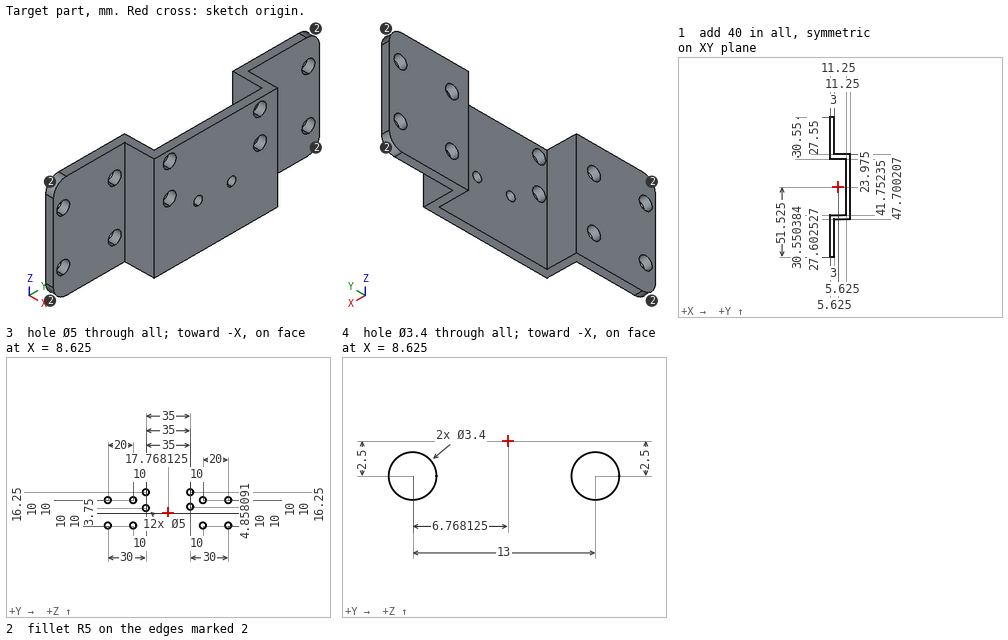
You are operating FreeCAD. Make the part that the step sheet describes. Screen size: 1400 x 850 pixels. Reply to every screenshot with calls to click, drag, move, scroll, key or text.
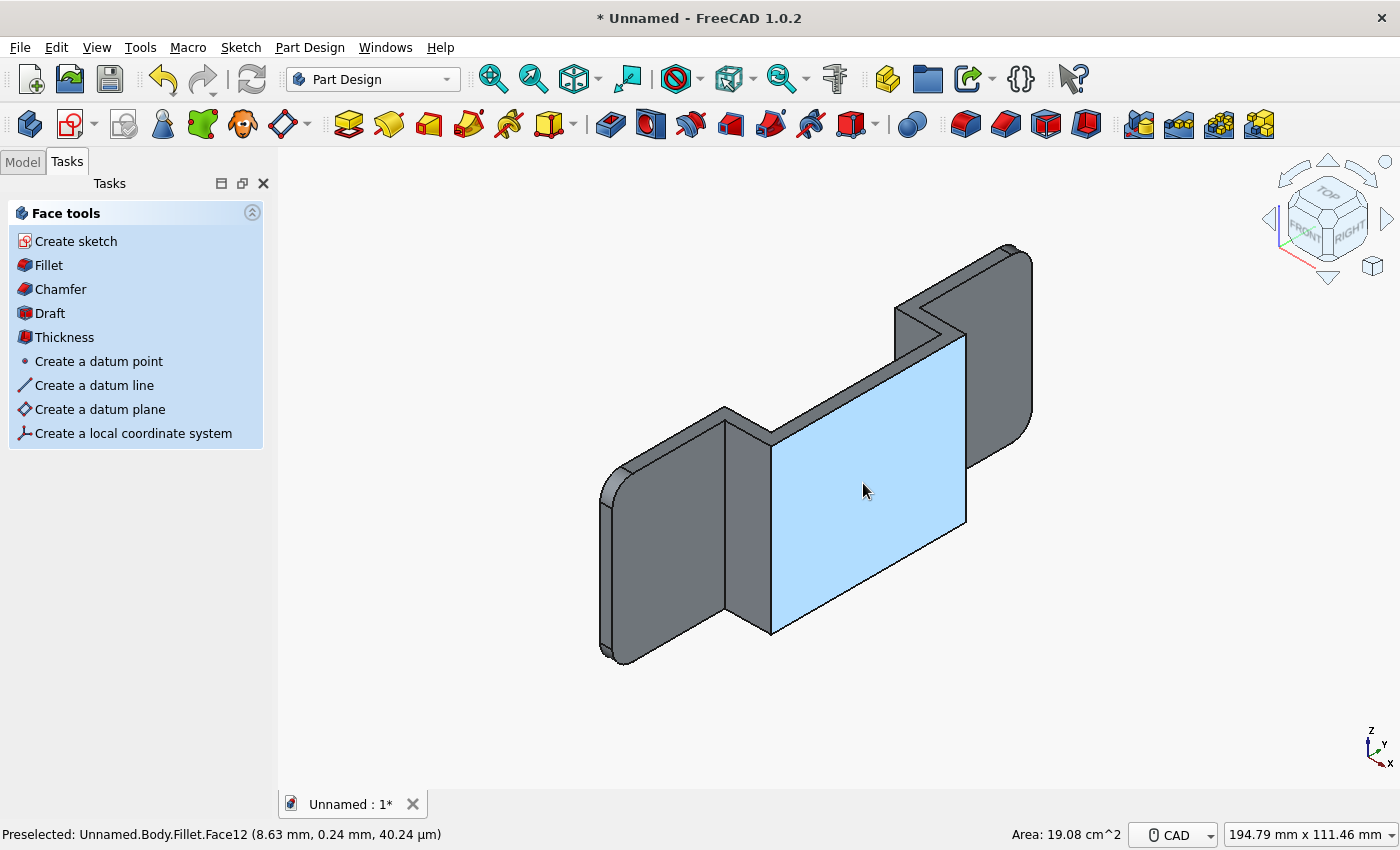
click(70, 124)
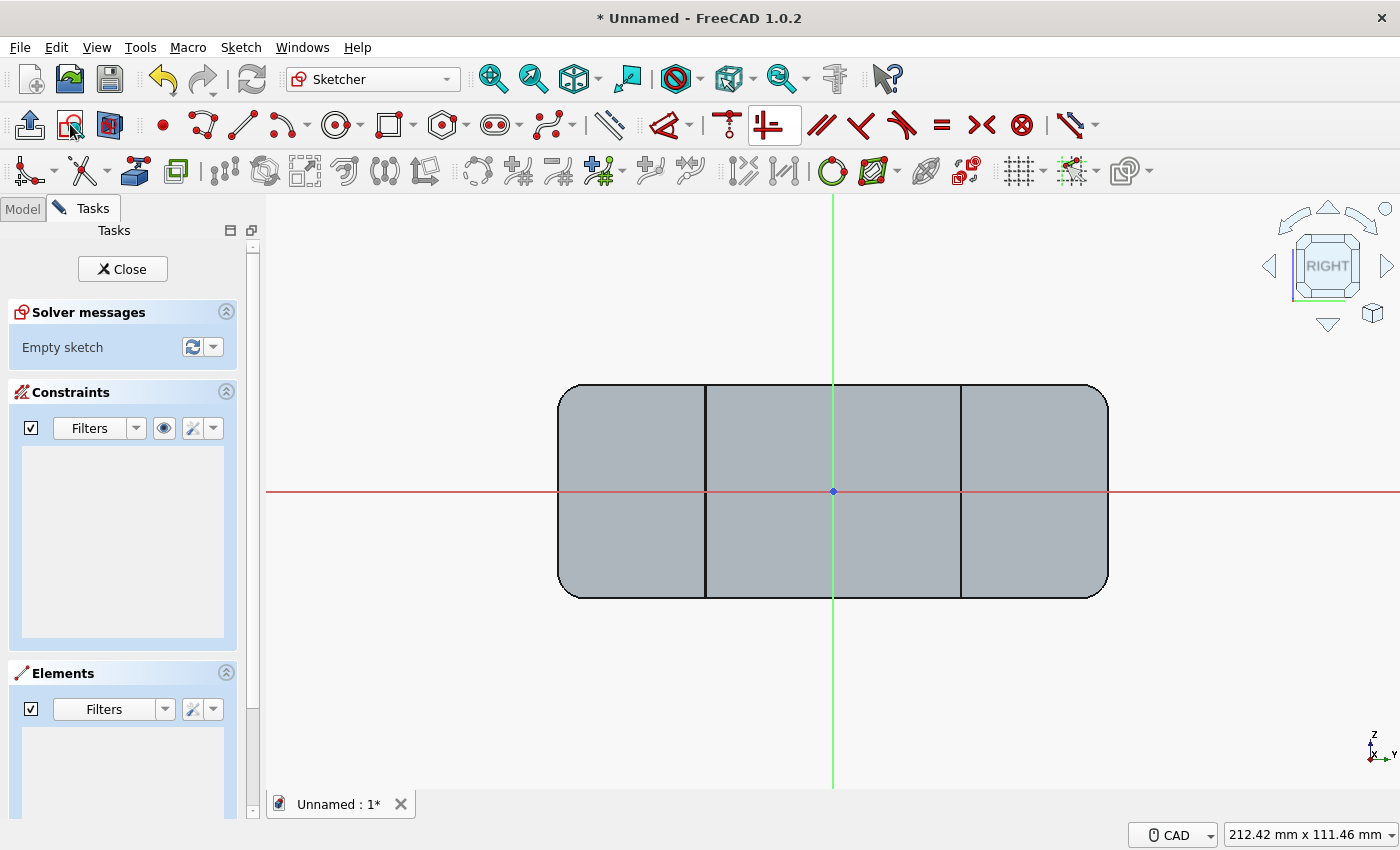
click(336, 126)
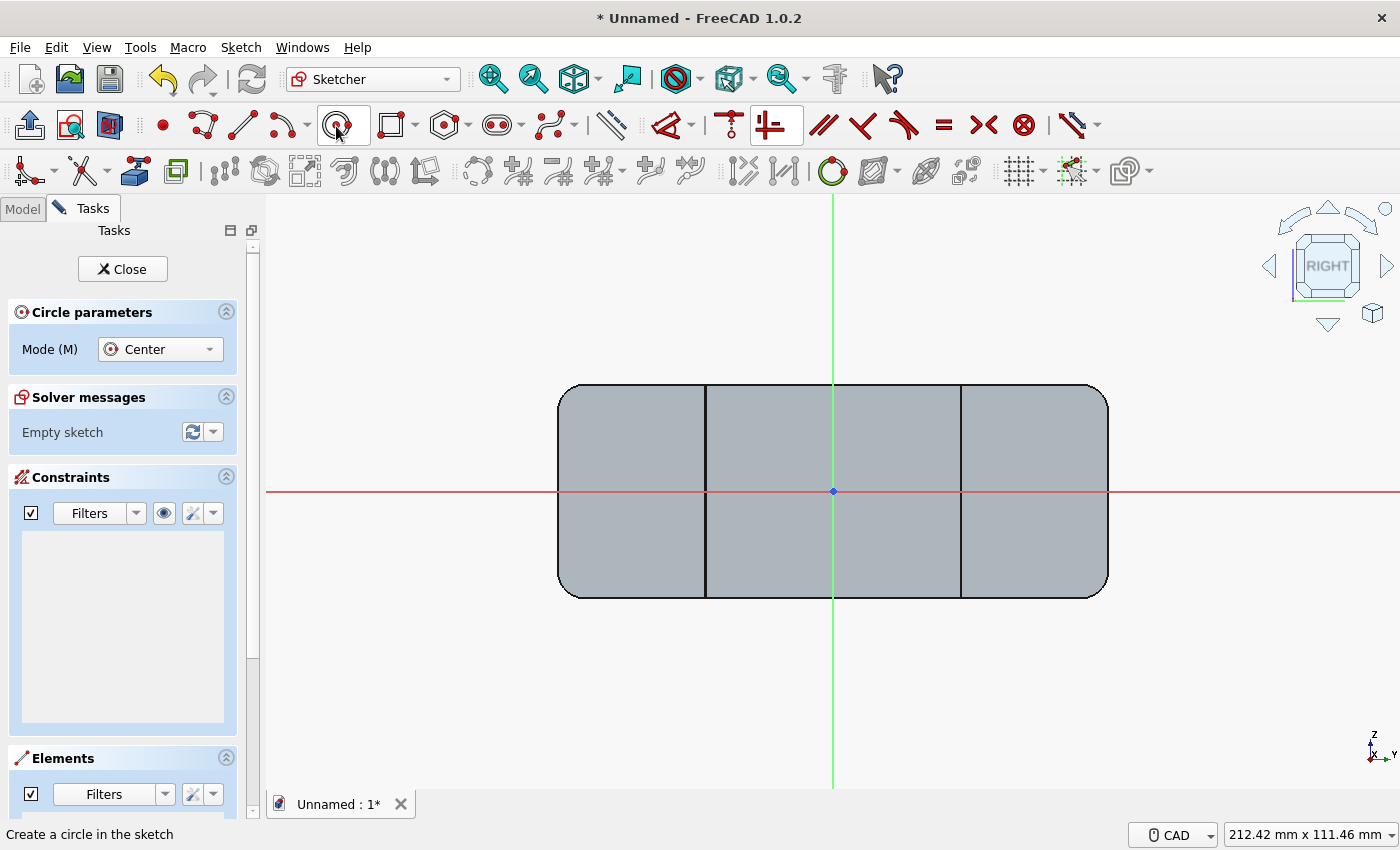
scroll(738, 471, up, 3)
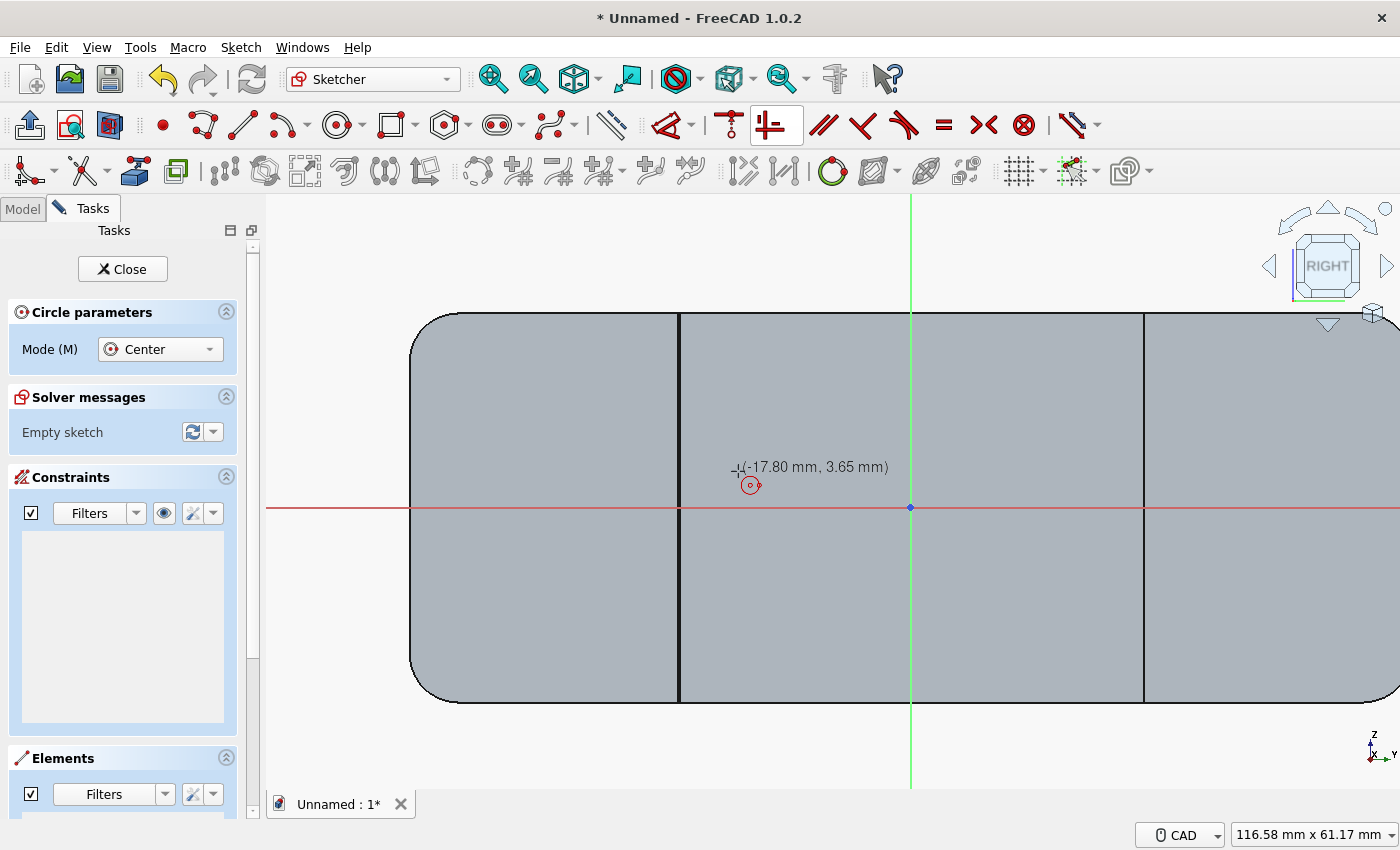
click(738, 471)
click(755, 454)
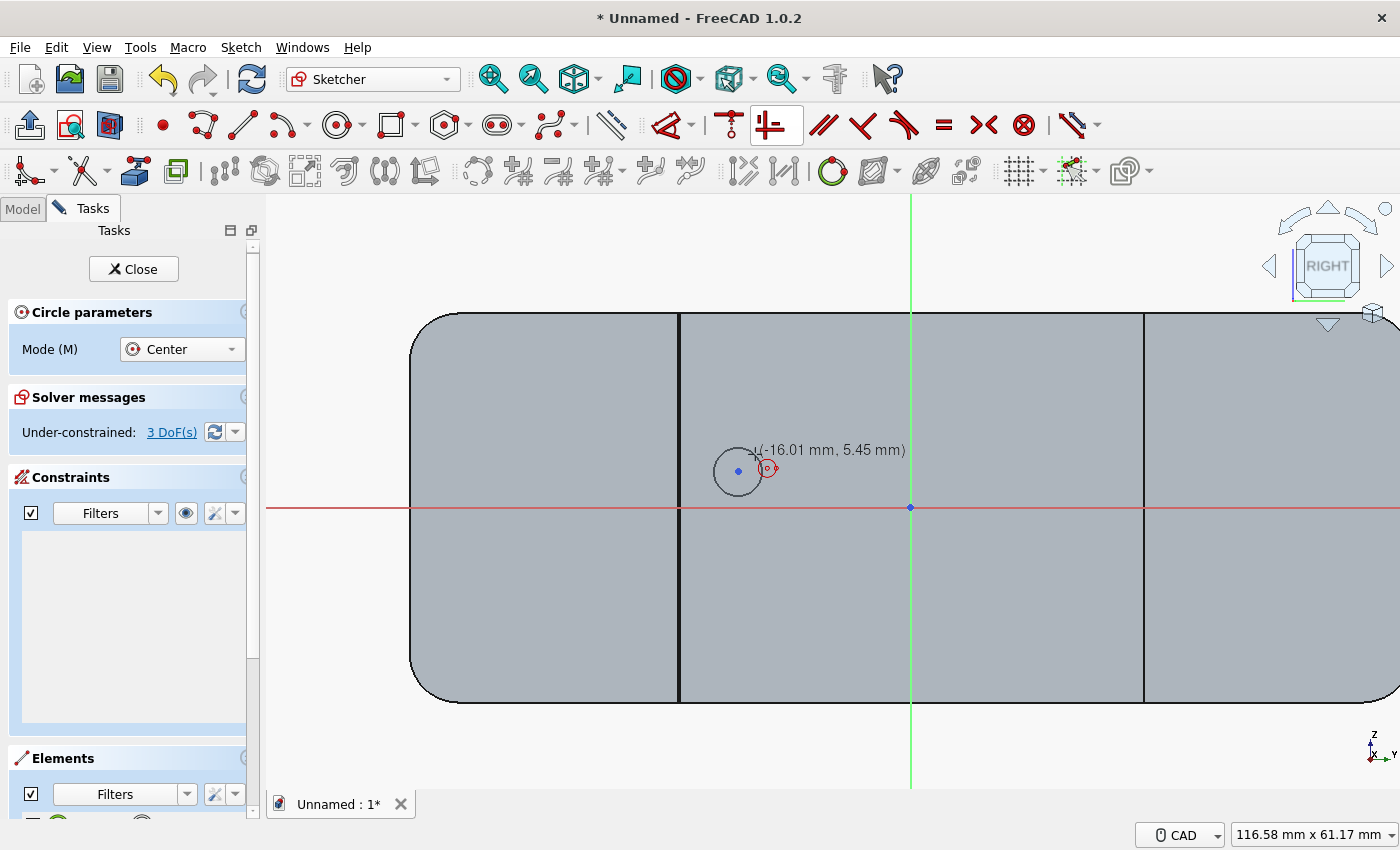
click(738, 350)
click(755, 333)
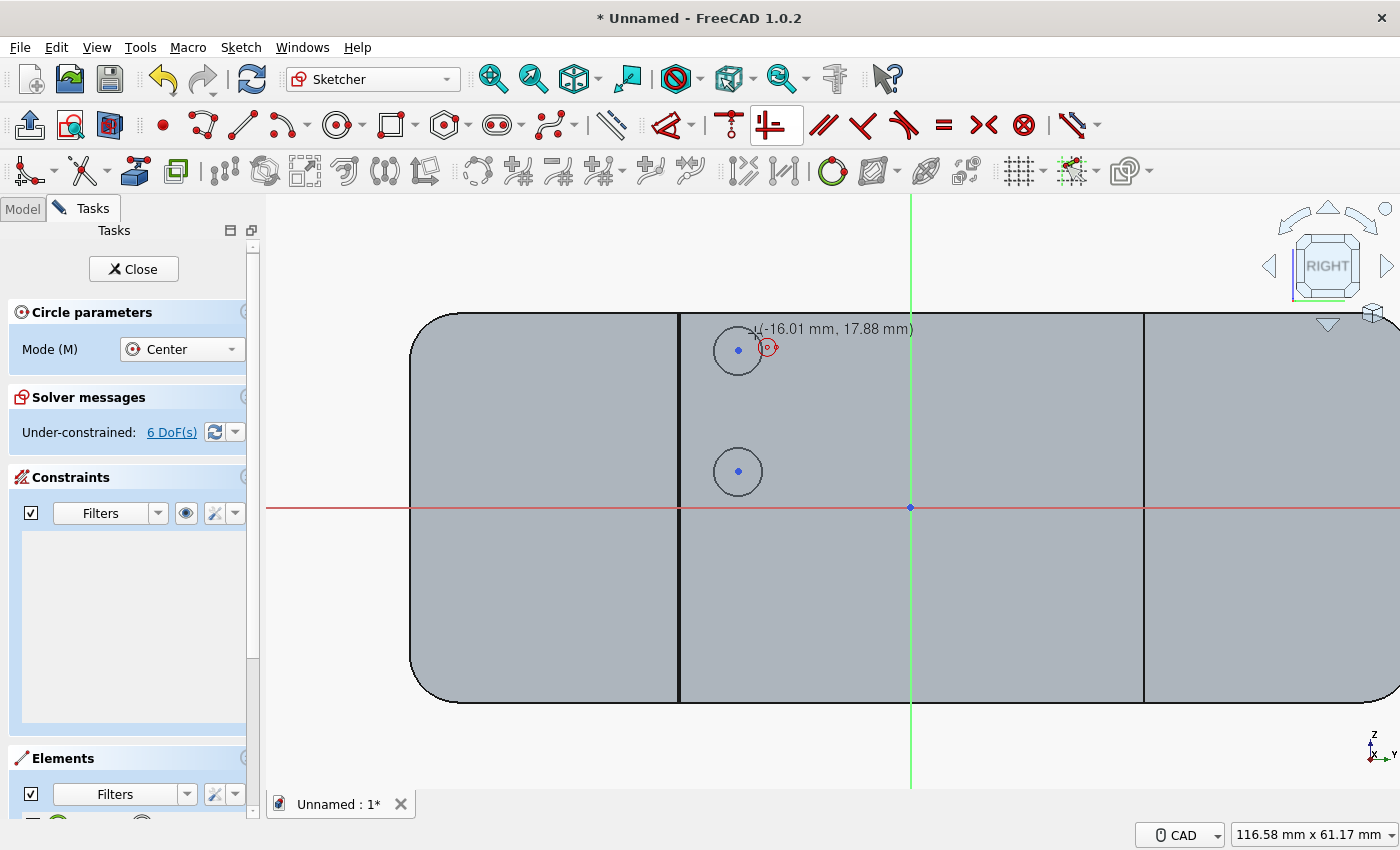
click(1078, 461)
click(1096, 444)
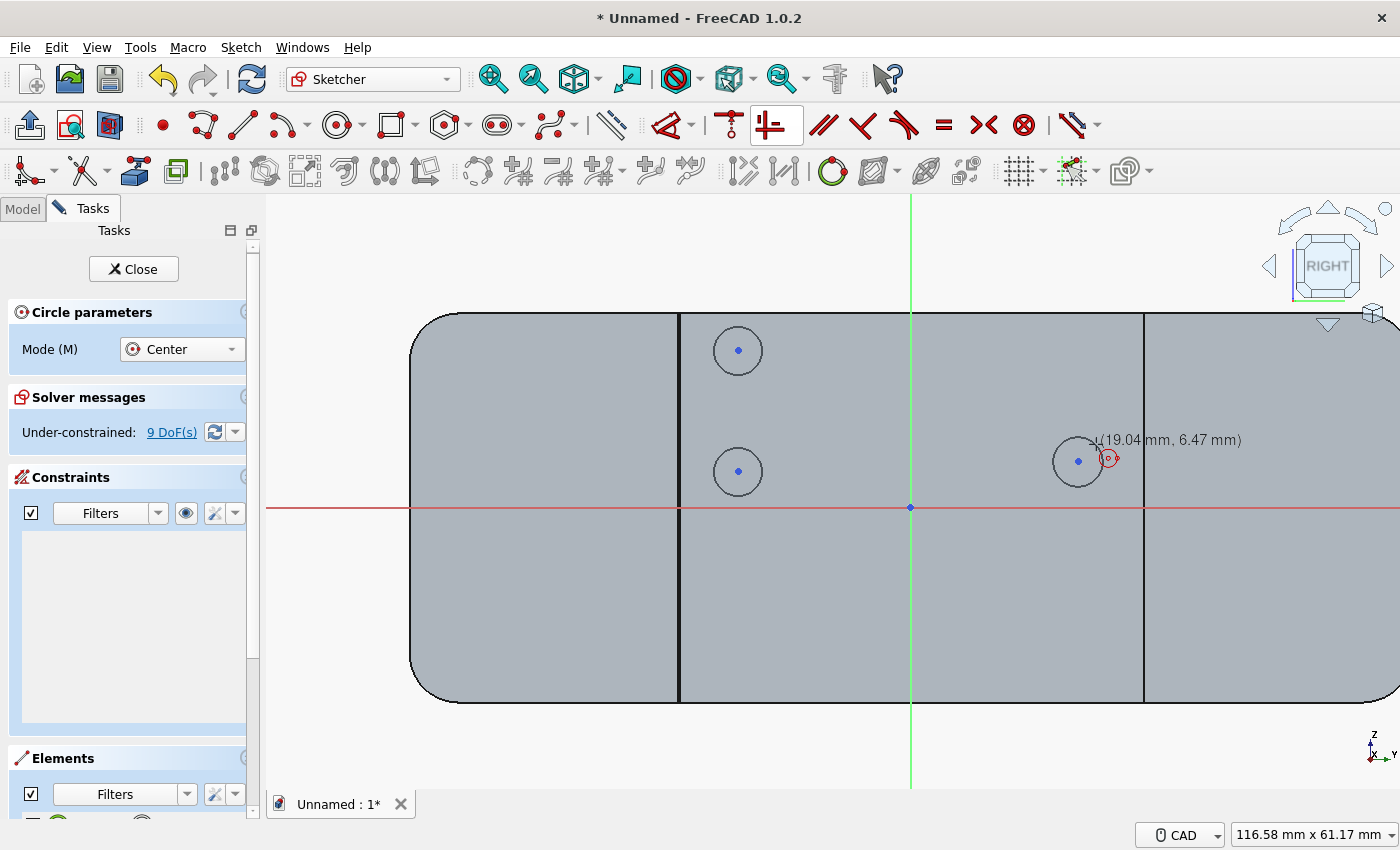
click(1078, 350)
click(1096, 333)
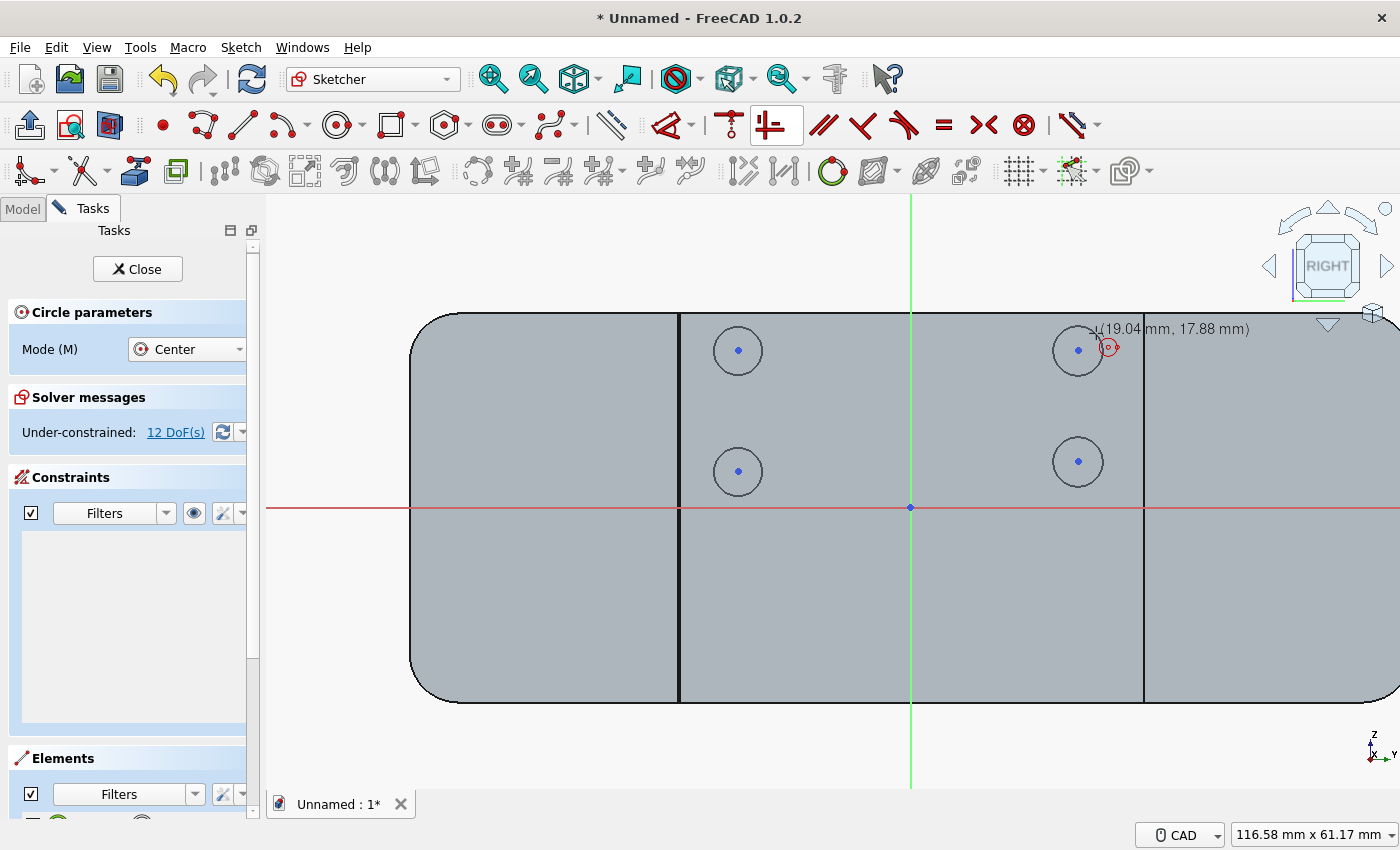
scroll(472, 520, down, 2)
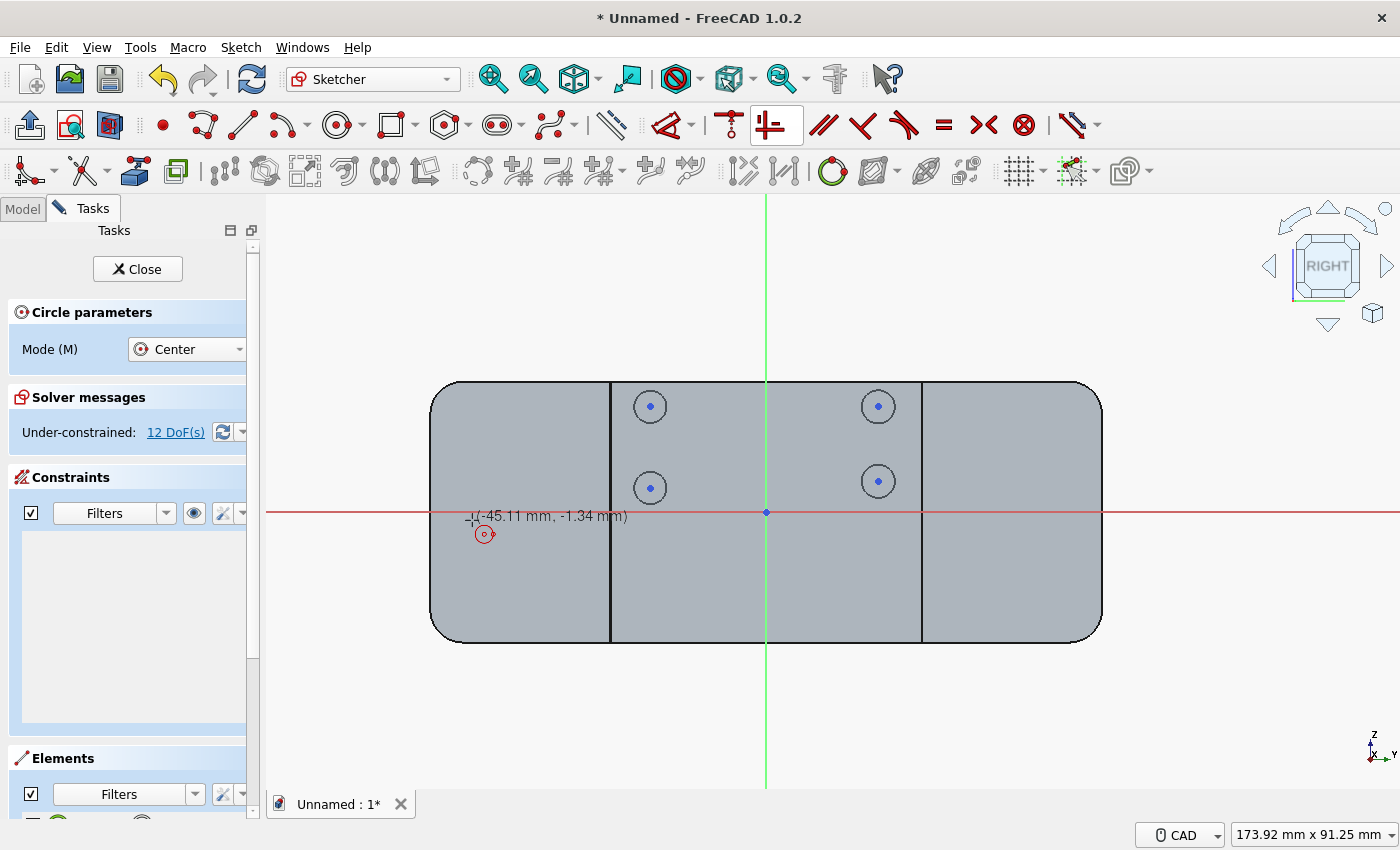
scroll(1074, 577, up, 2)